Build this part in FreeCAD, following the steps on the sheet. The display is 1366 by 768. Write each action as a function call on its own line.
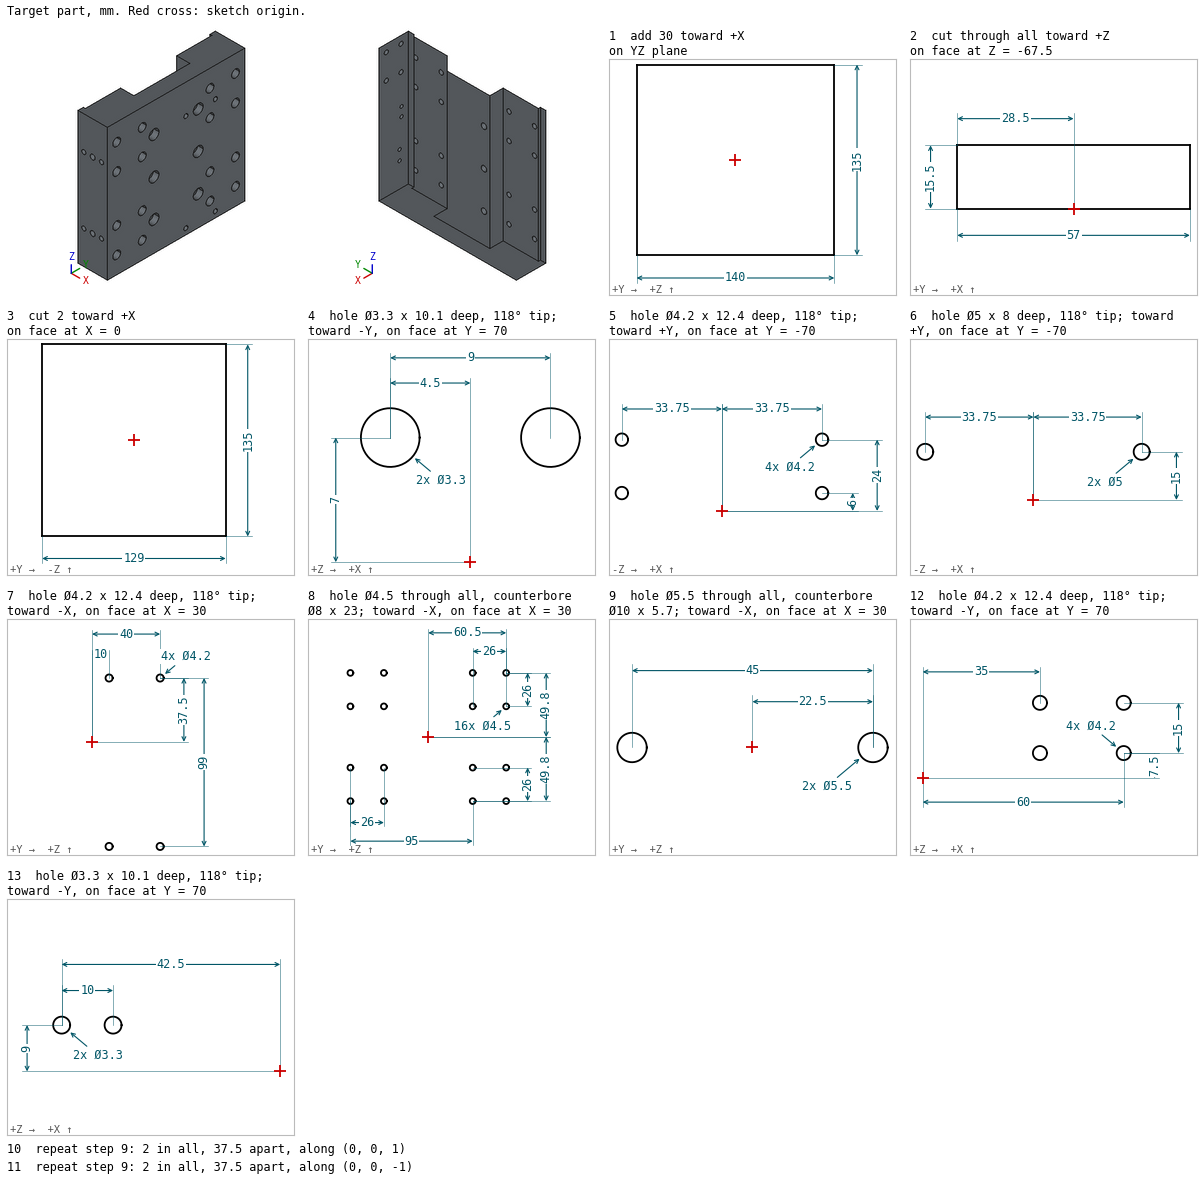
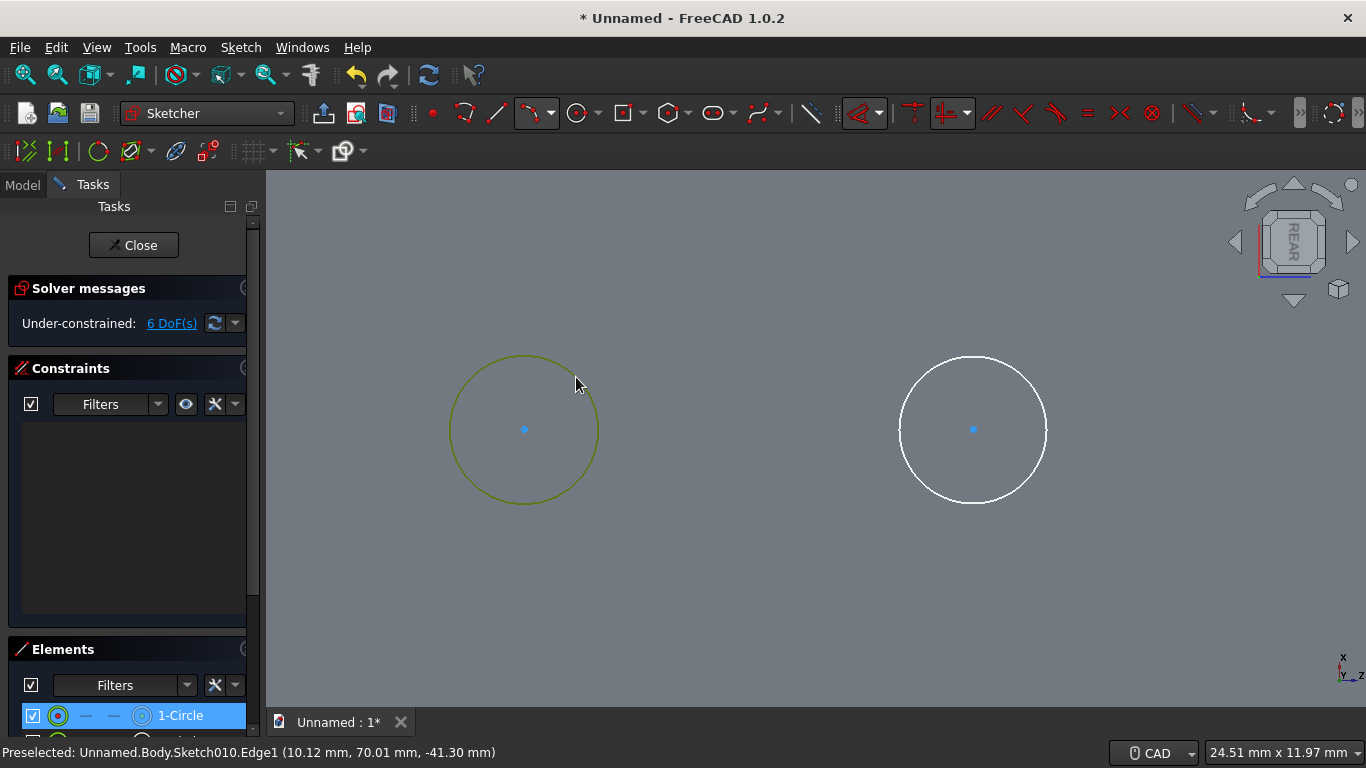
click(1025, 378)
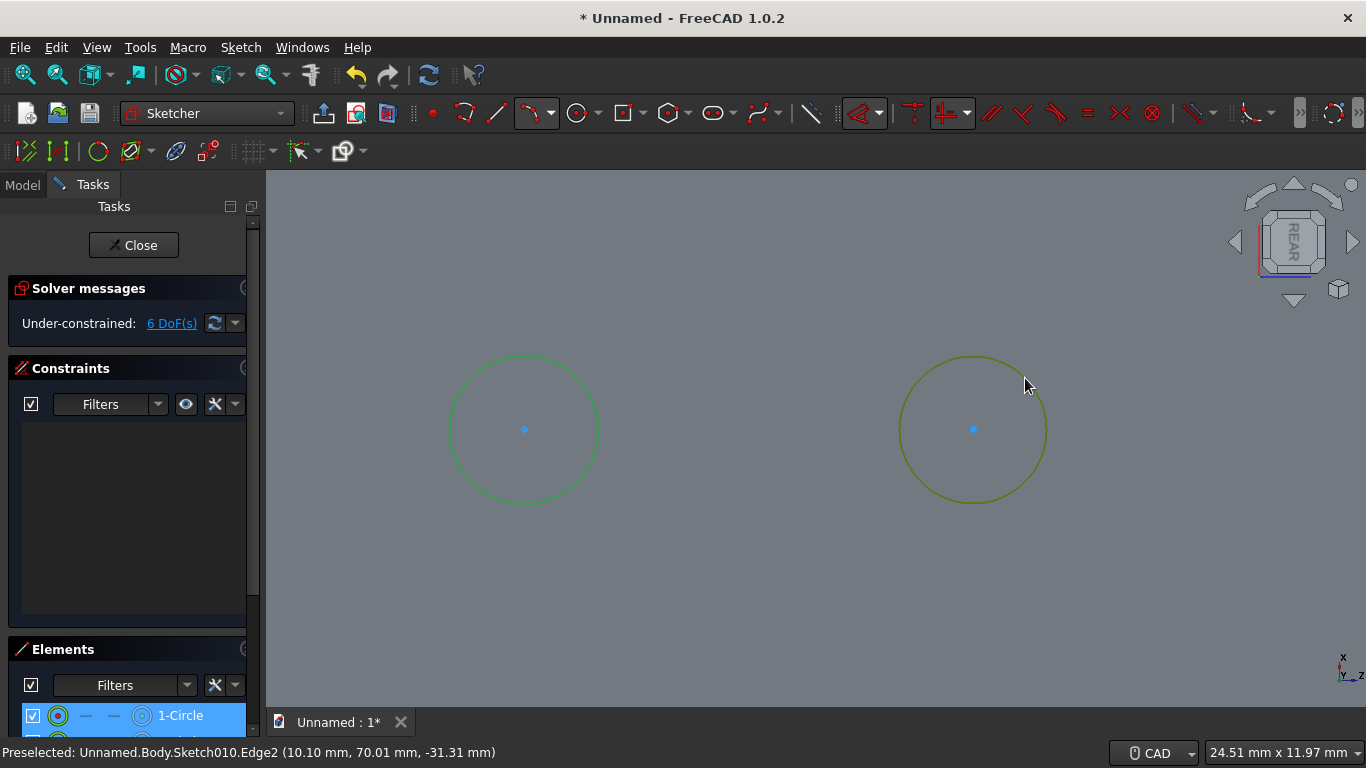
click(1088, 114)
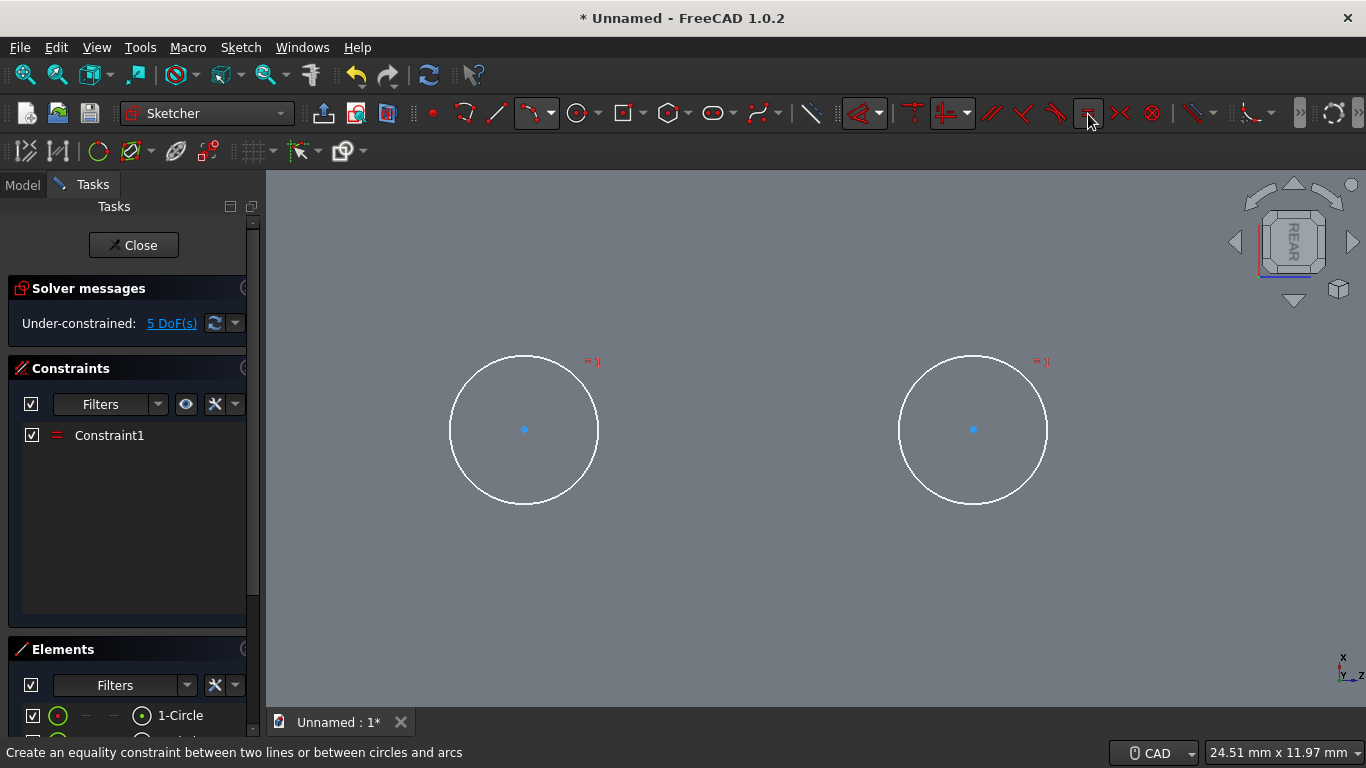
click(524, 430)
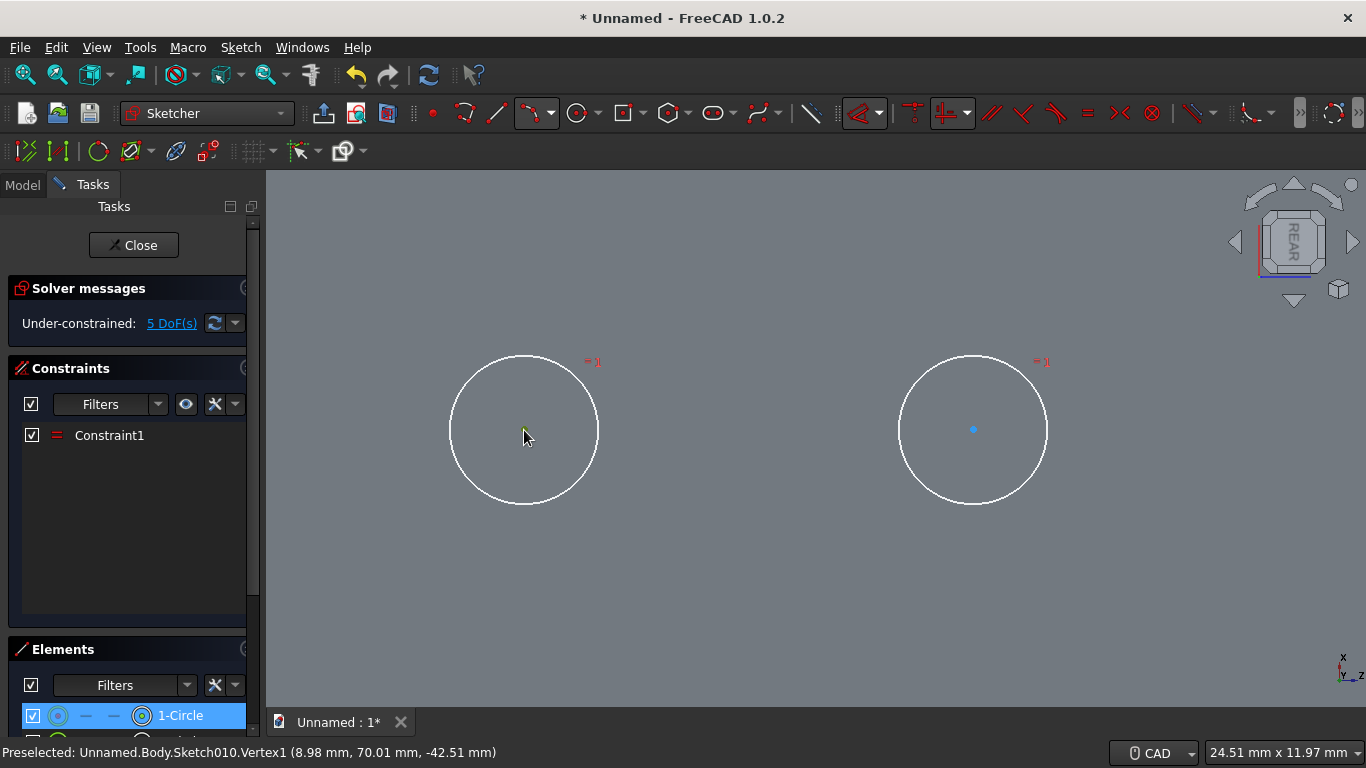
click(973, 430)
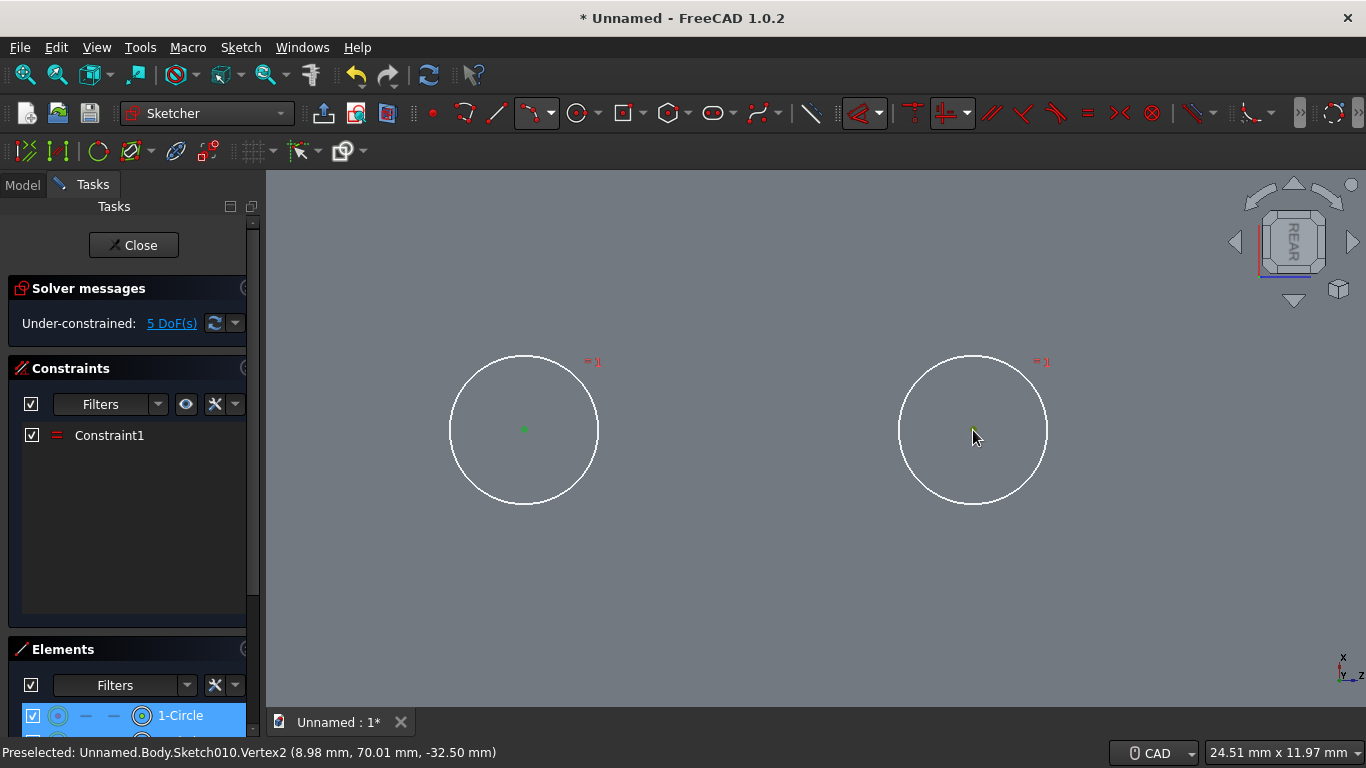
key(h)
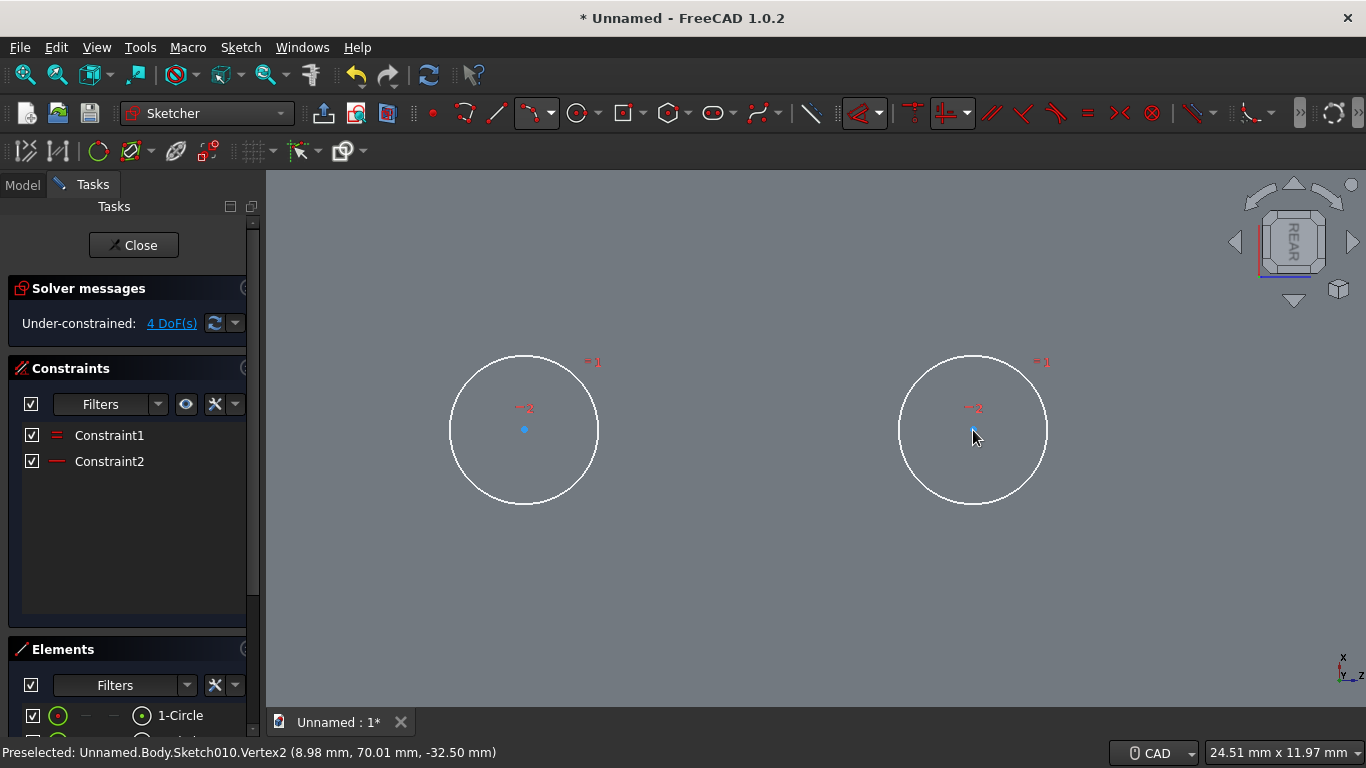
click(576, 377)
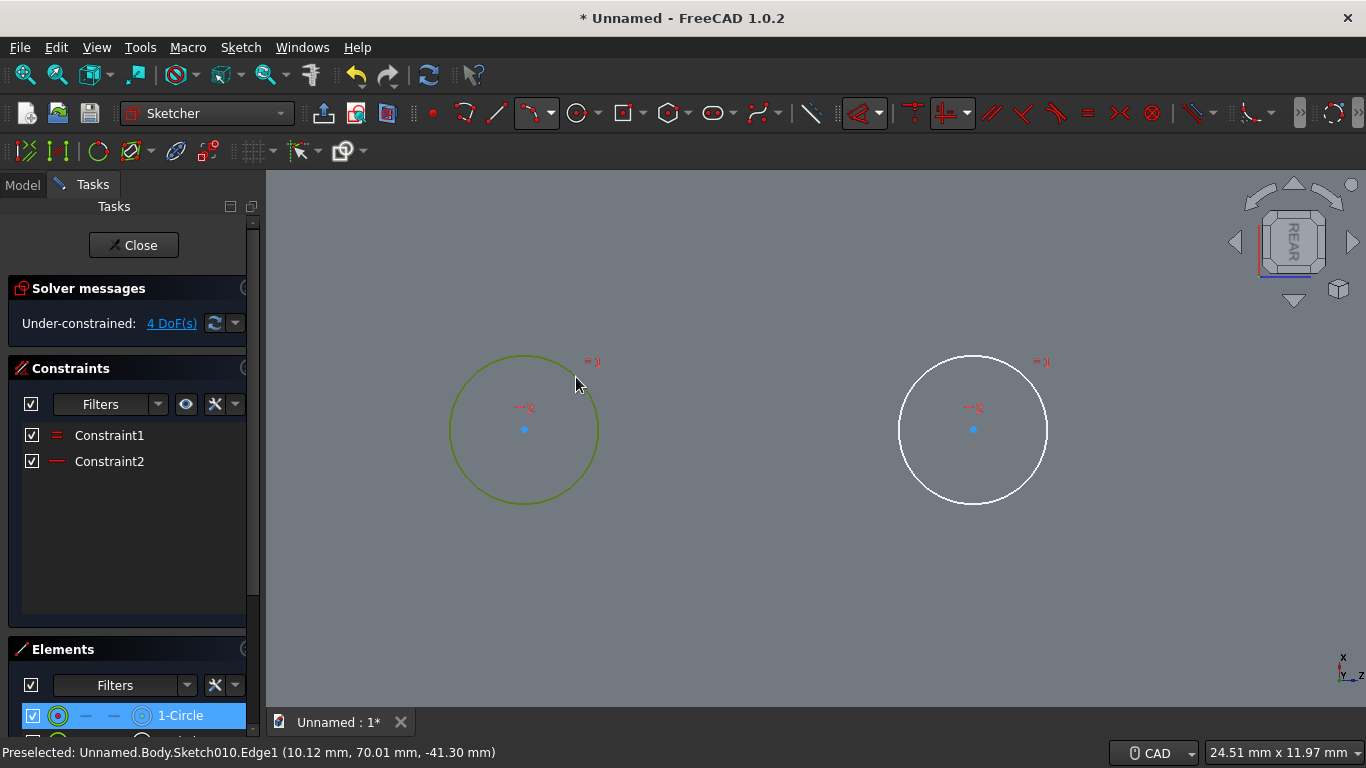
click(882, 114)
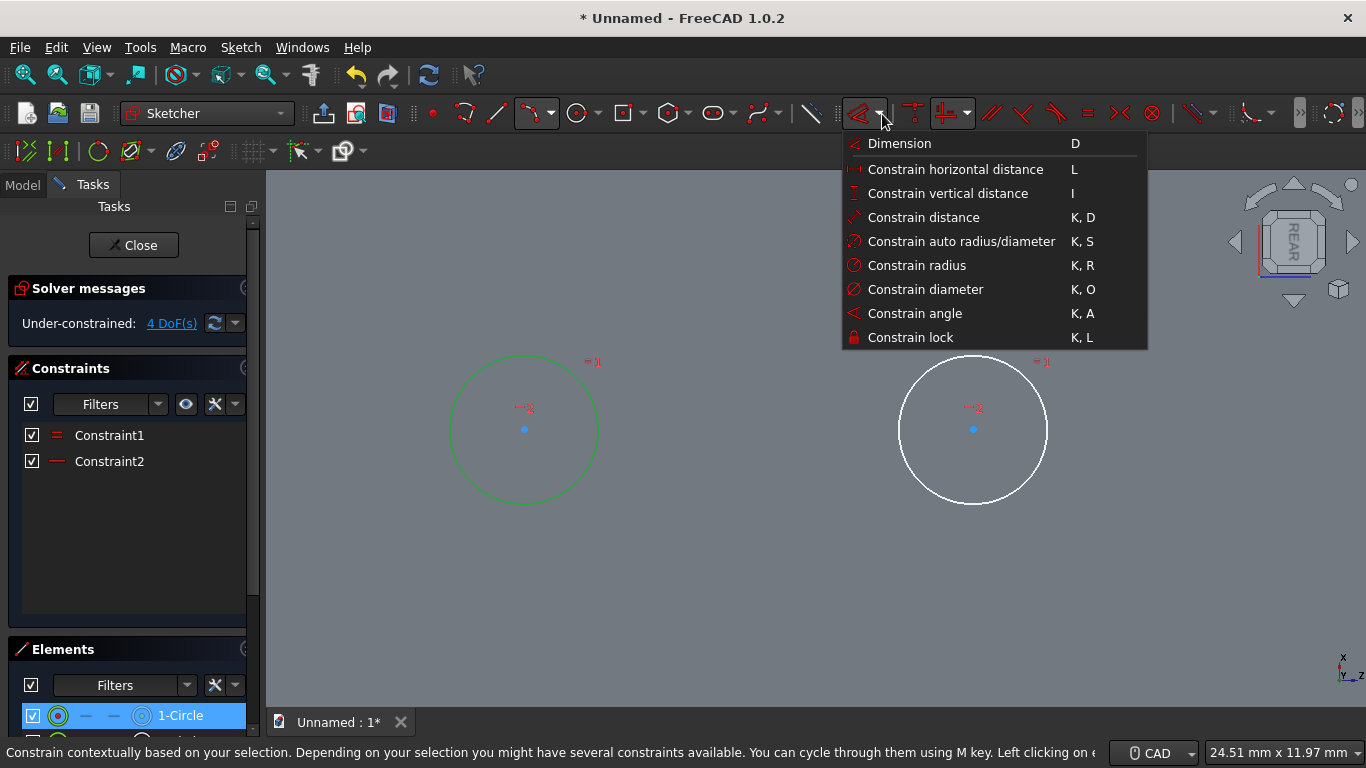
click(995, 289)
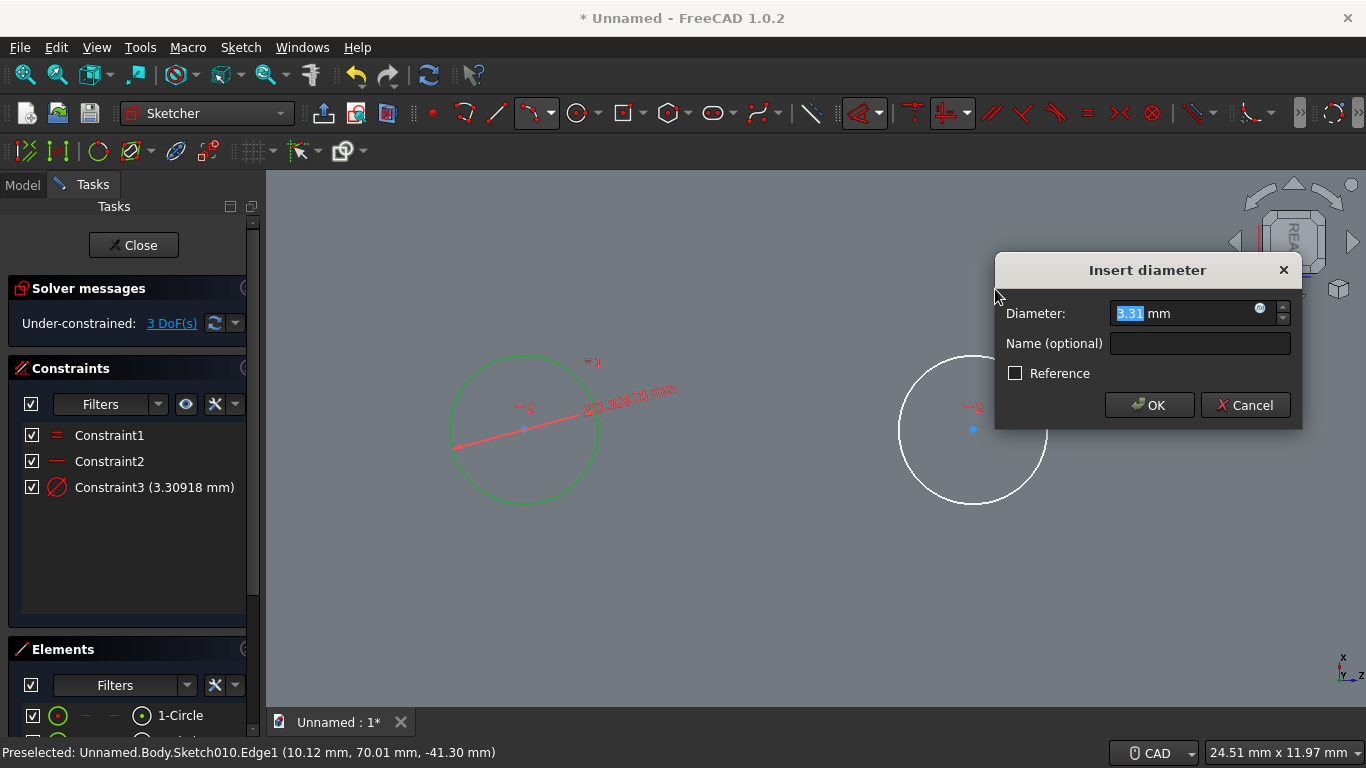
text(3.3)
key(Return)